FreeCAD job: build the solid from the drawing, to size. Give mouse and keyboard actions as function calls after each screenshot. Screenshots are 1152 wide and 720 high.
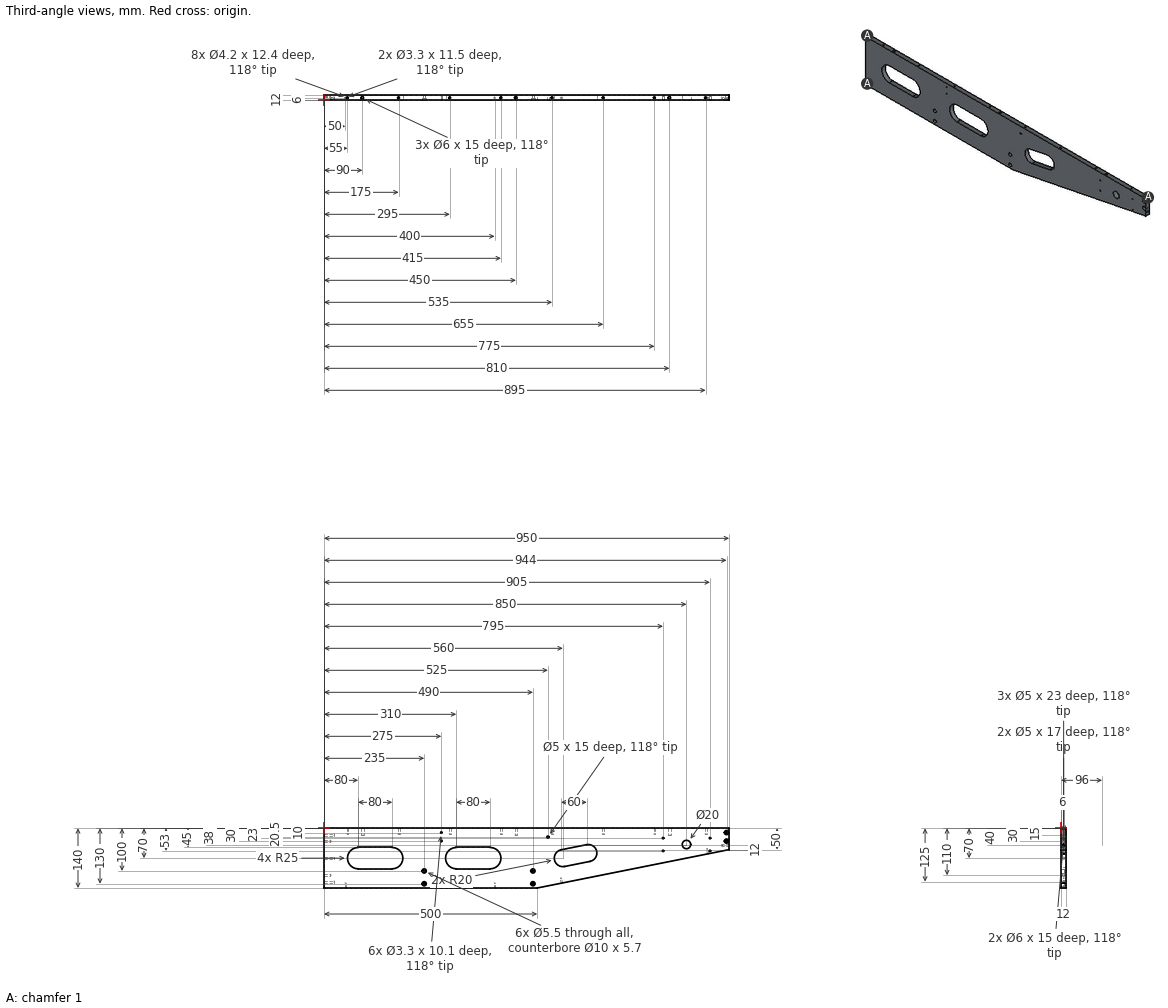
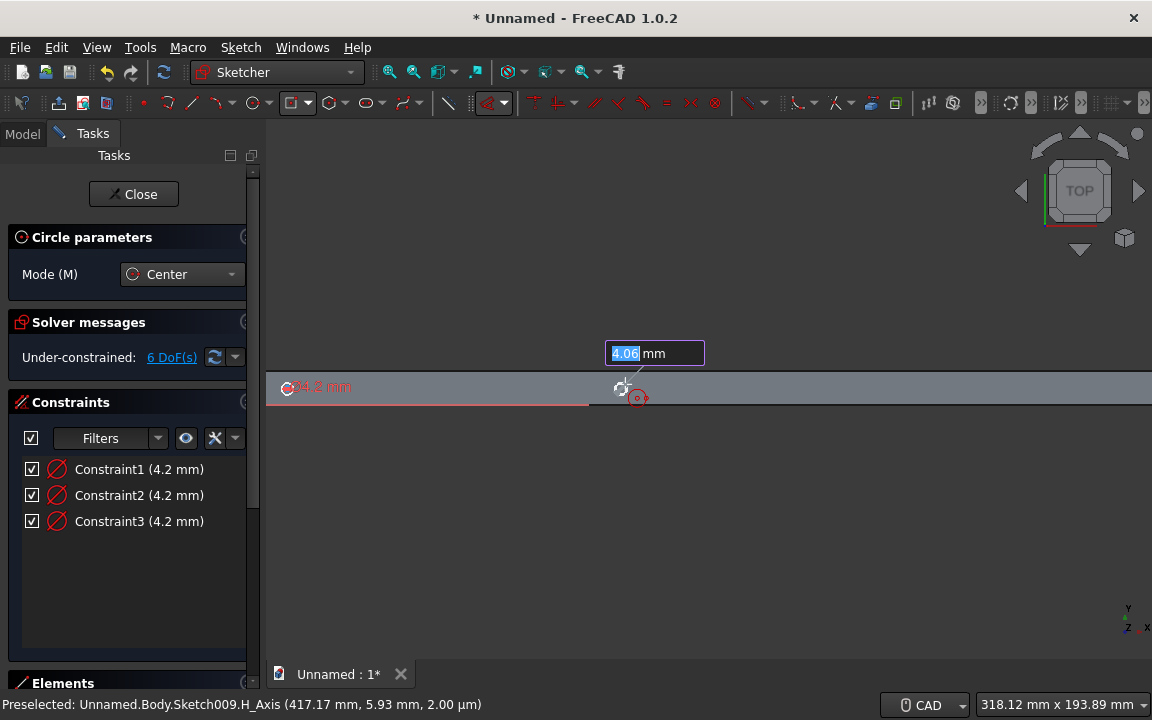
text(4.2)
key(Return)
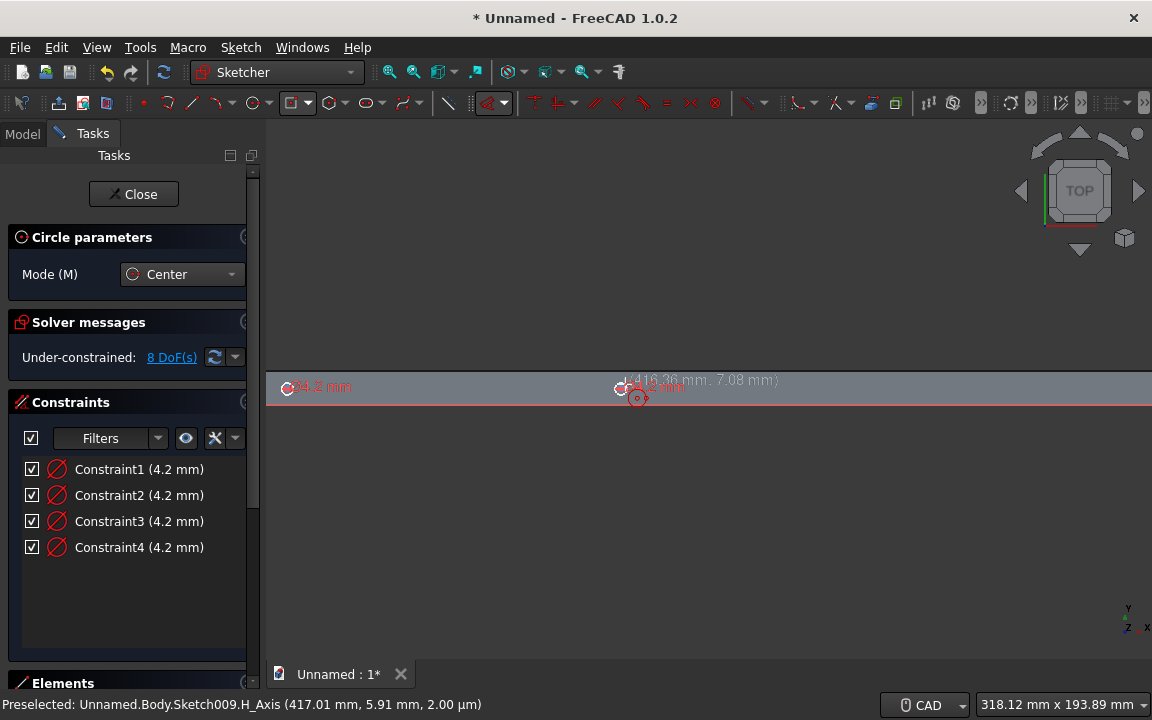
scroll(955, 388, up, 7)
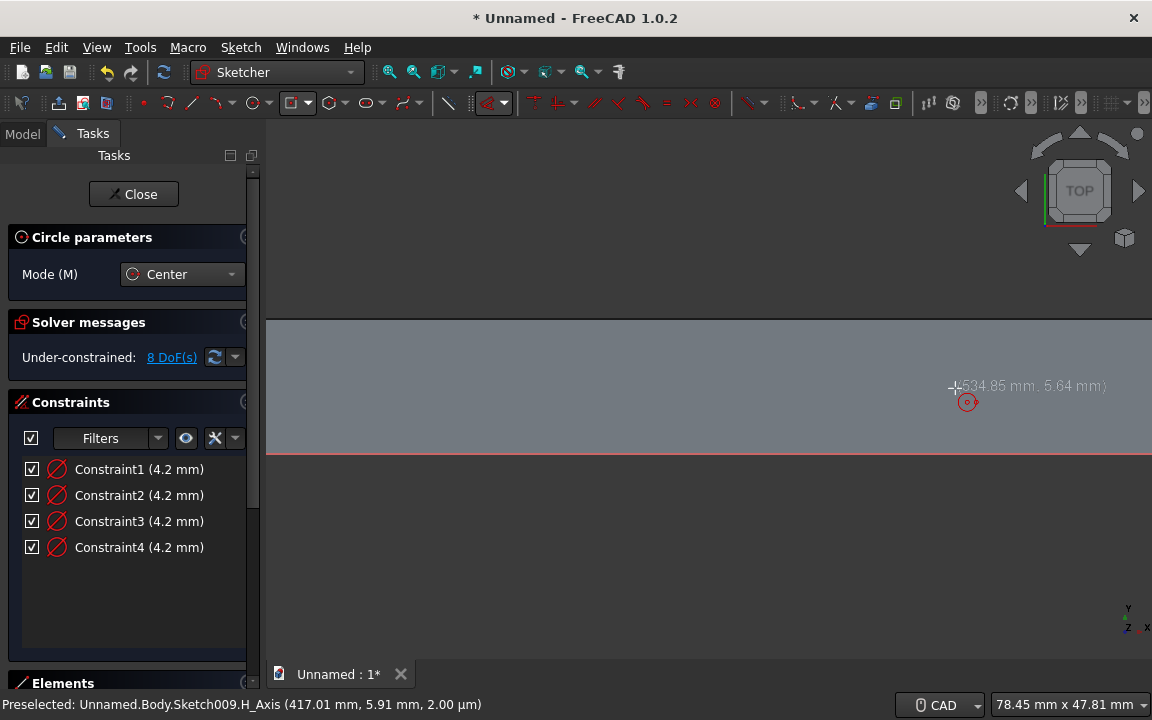
scroll(675, 388, down, 15)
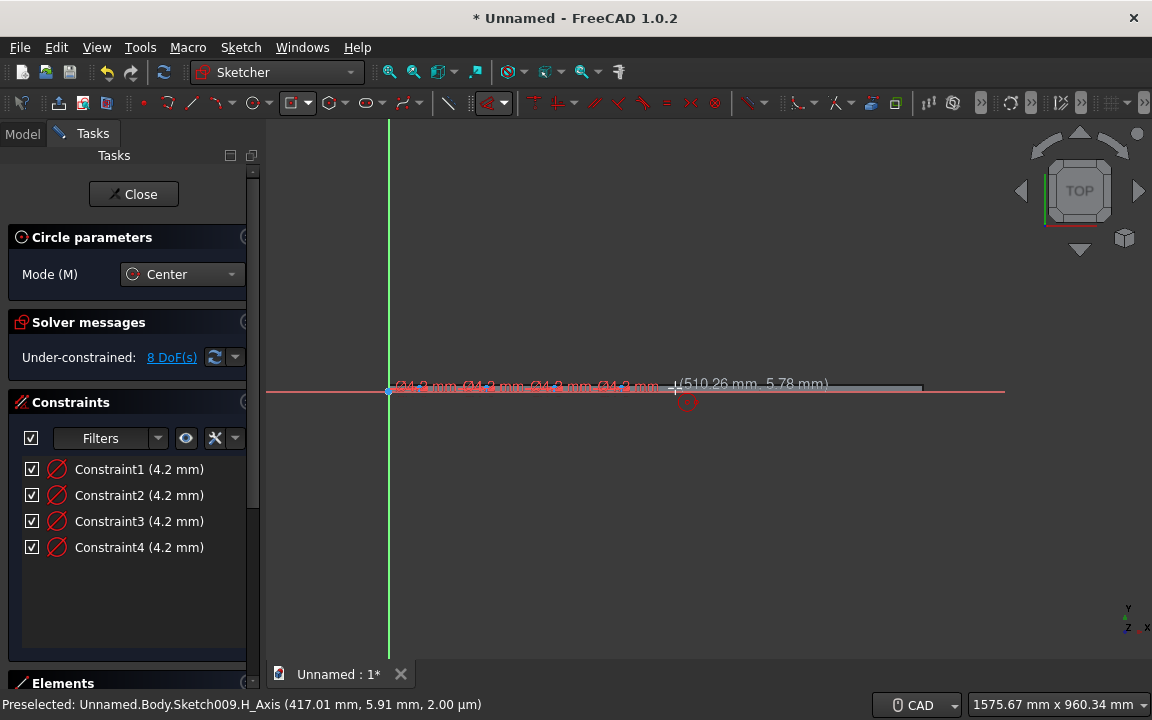
scroll(689, 388, up, 8)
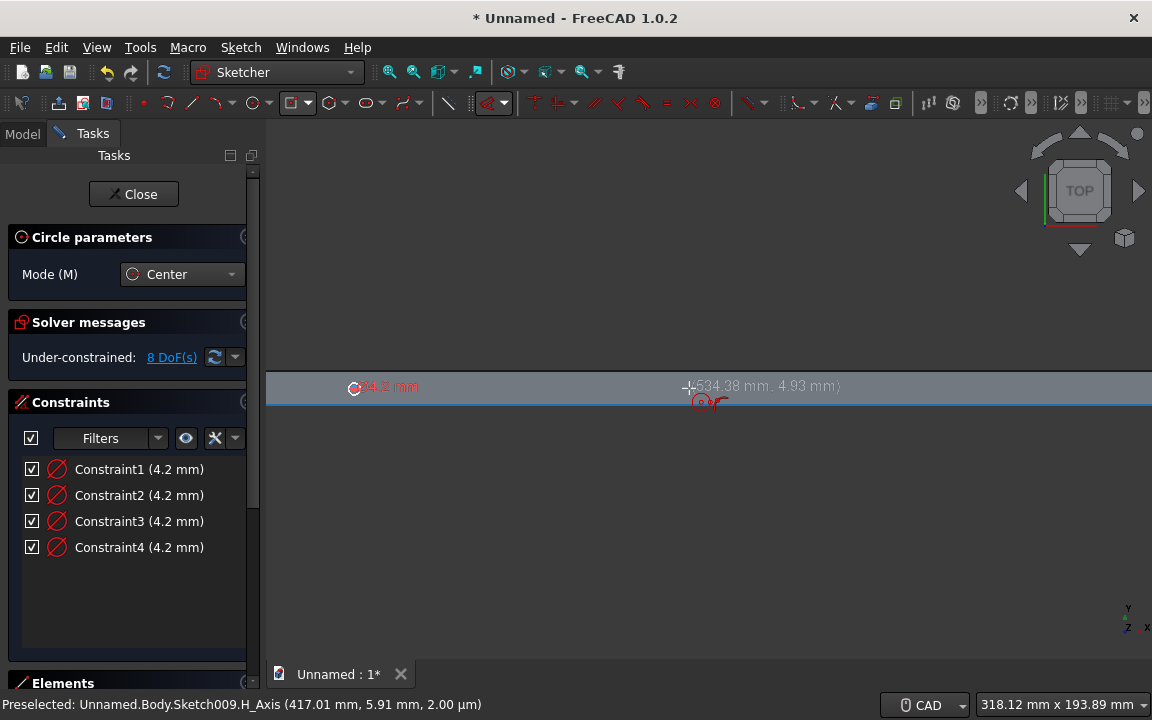
click(689, 388)
move(693, 384)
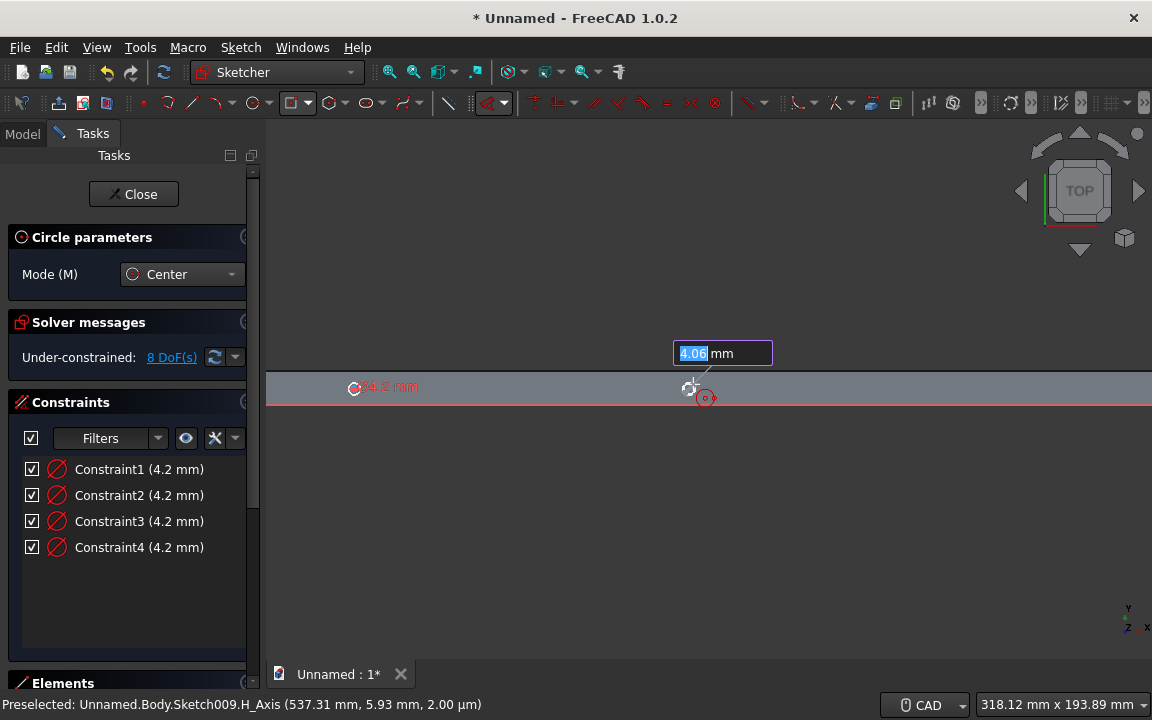
text(4.2)
key(Return)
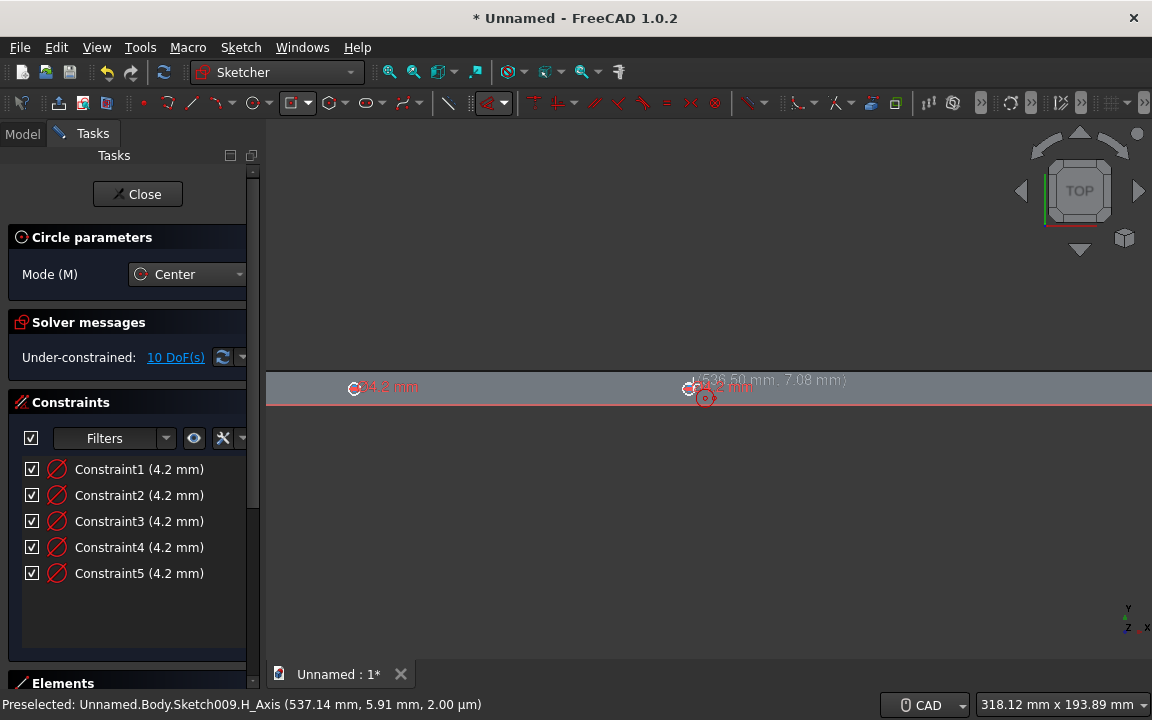
scroll(689, 388, down, 8)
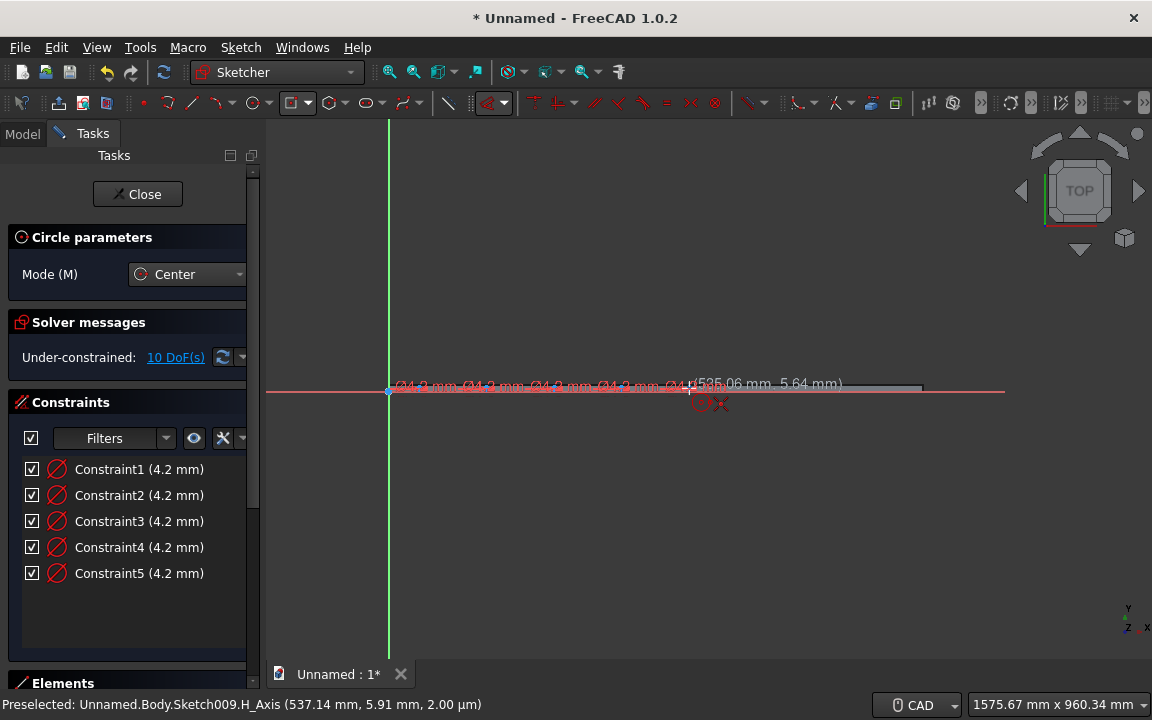
scroll(757, 388, up, 15)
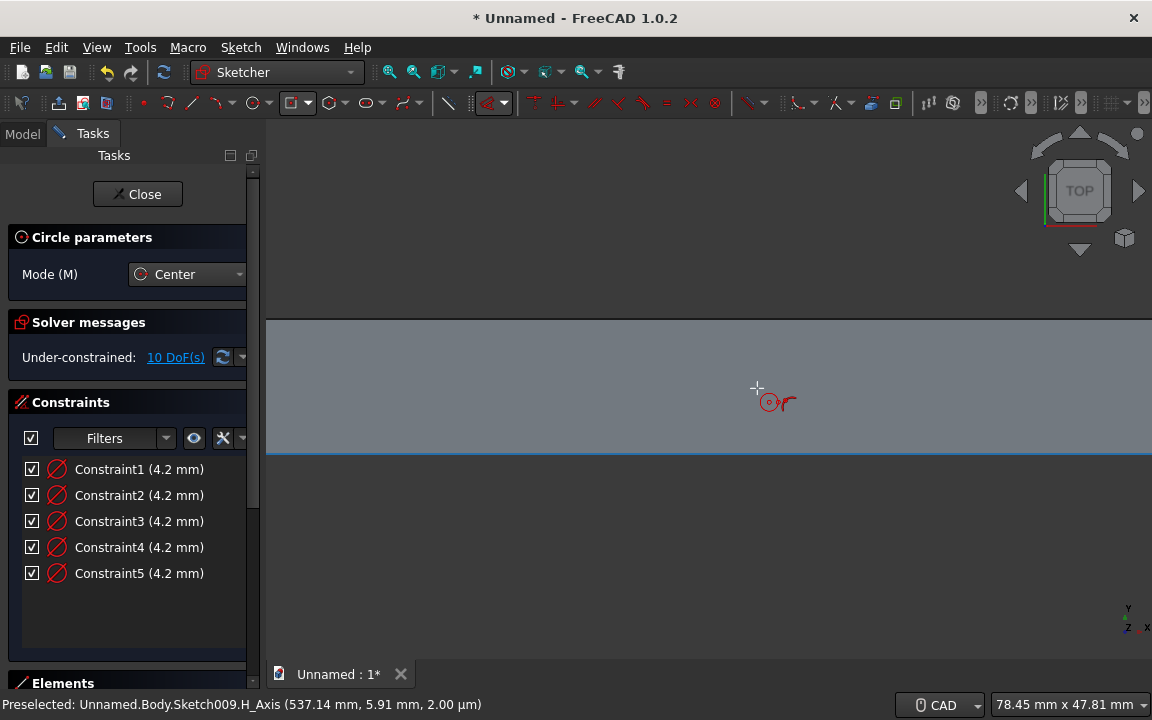
scroll(757, 388, down, 15)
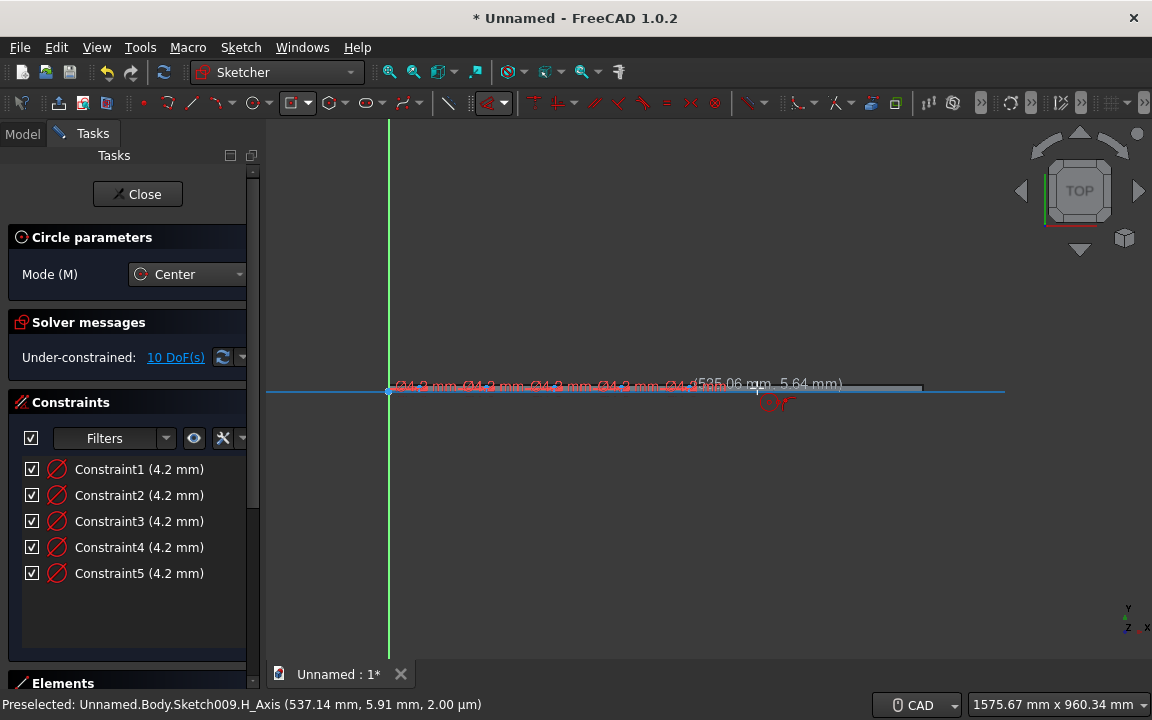
scroll(757, 388, up, 8)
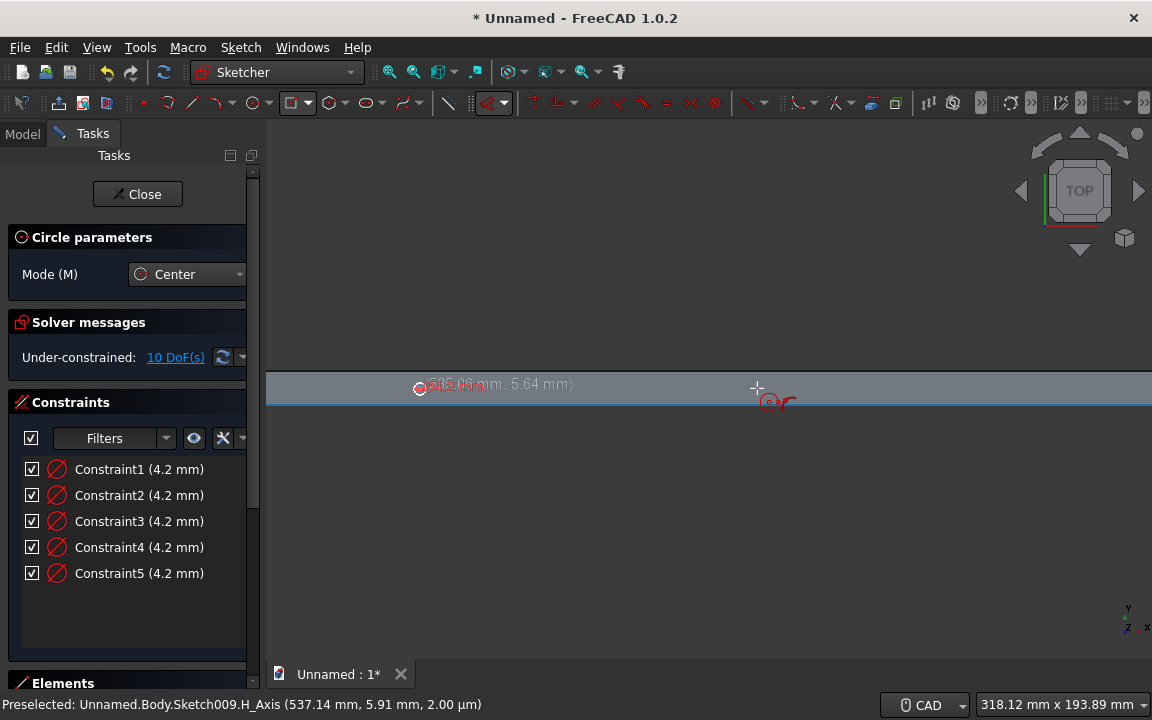
click(754, 388)
move(758, 384)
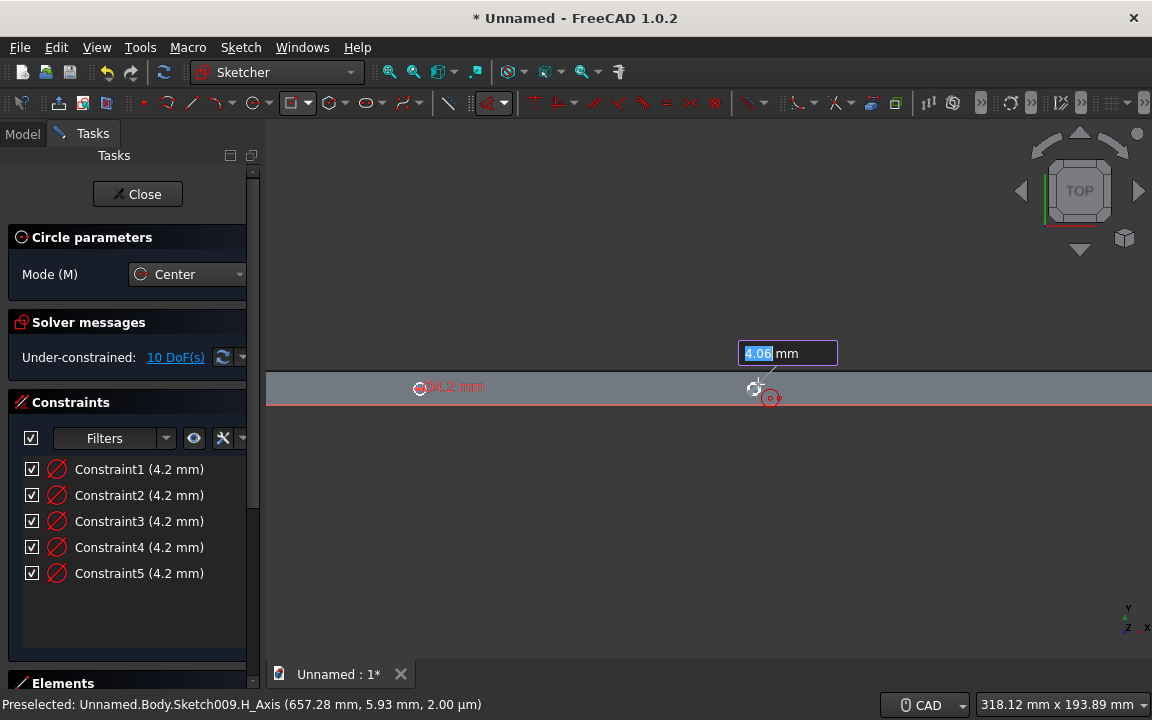
text(4.2)
key(Return)